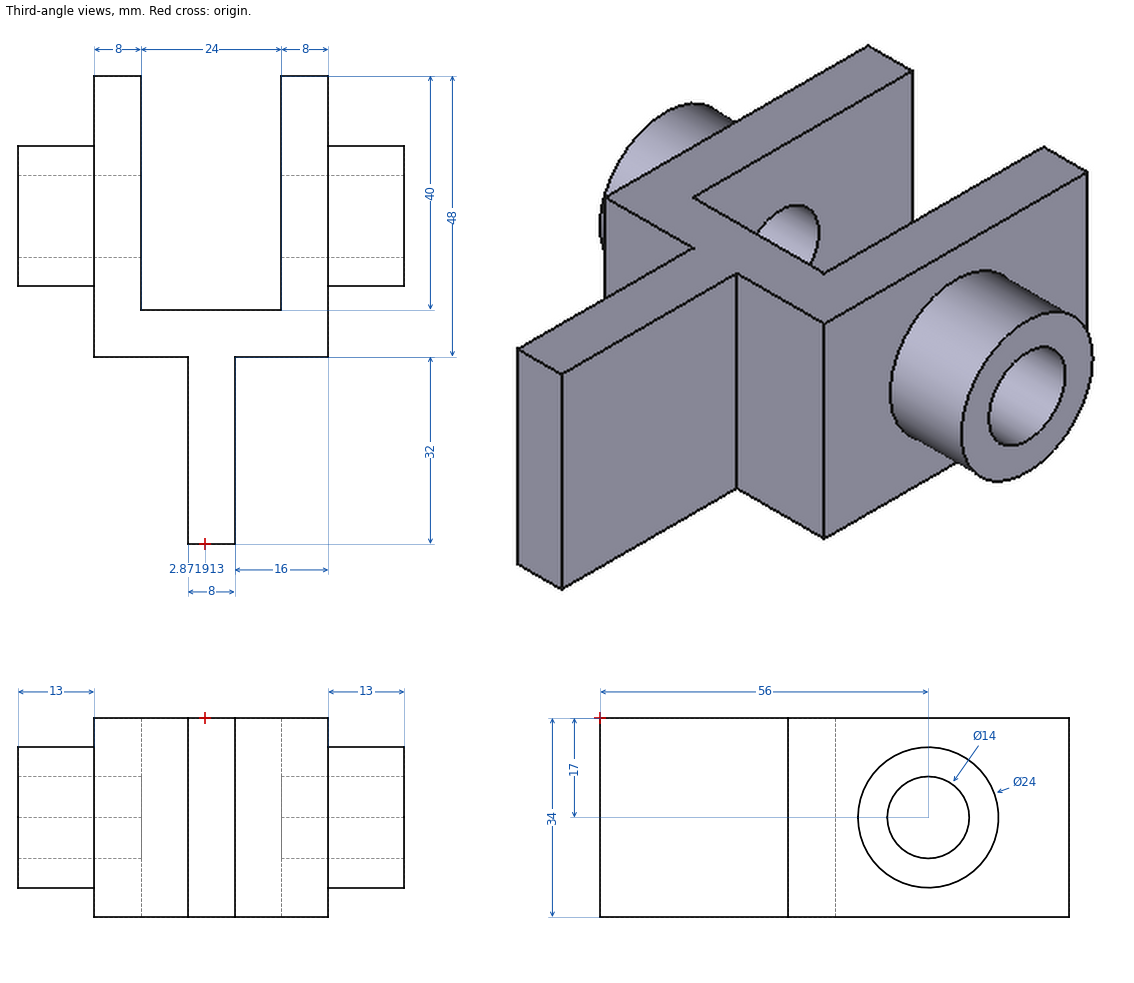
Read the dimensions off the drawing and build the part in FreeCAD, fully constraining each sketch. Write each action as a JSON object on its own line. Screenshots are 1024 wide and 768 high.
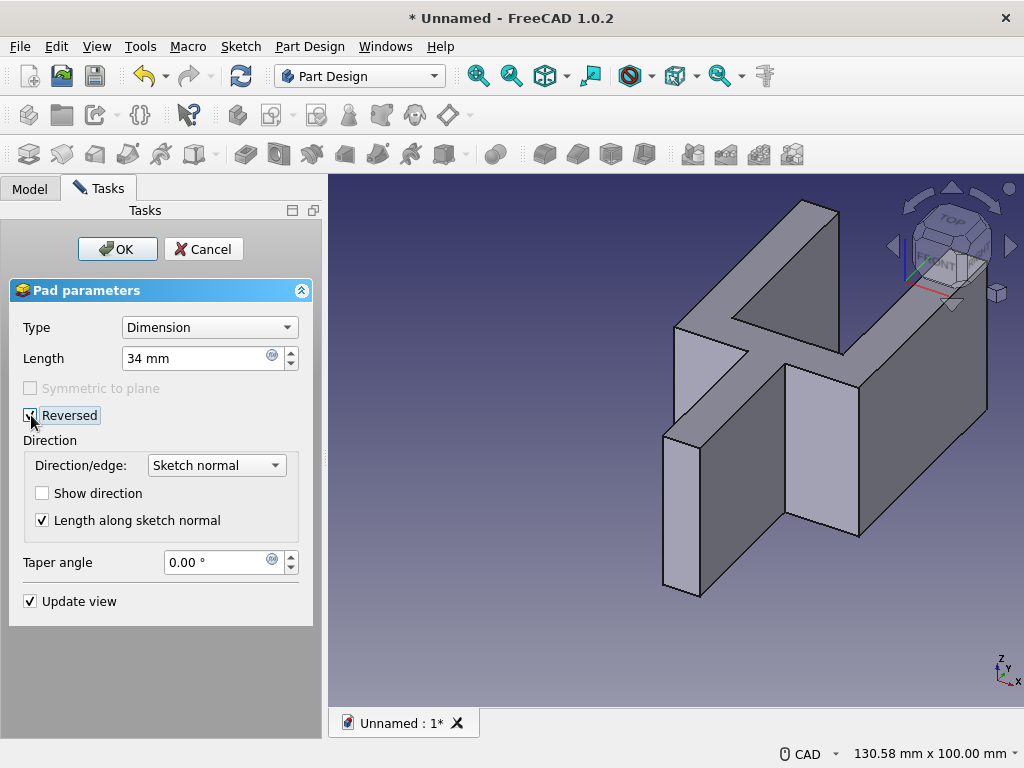
{"action": "left_click", "coordinate": [118, 249]}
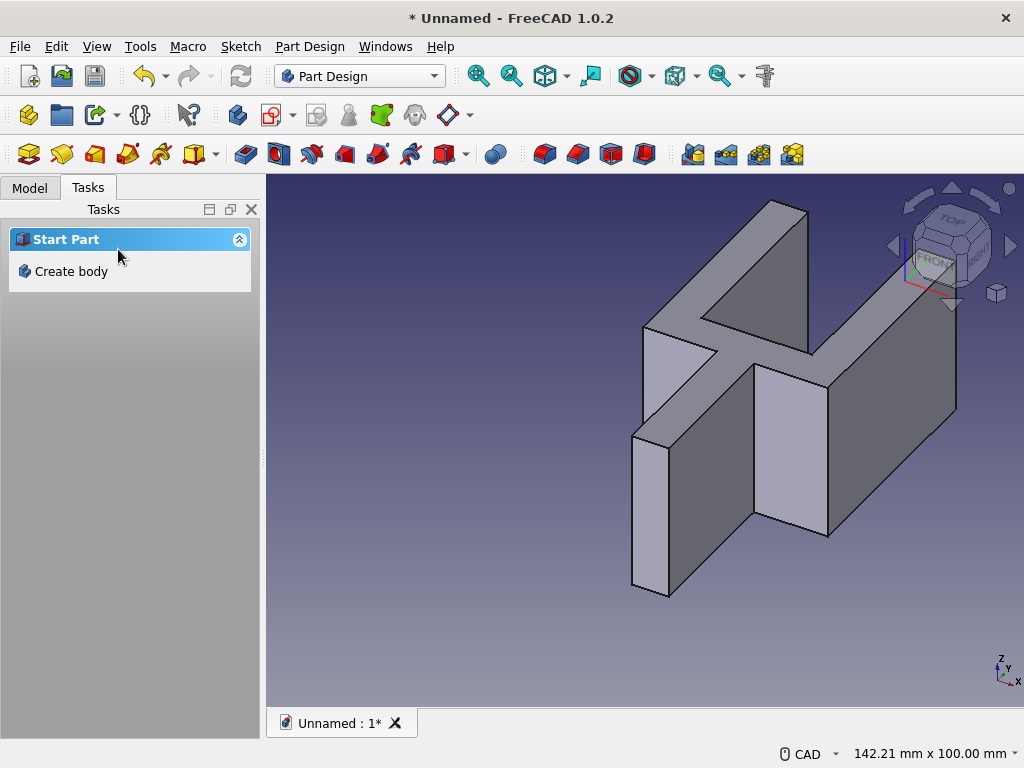
{"action": "left_click", "coordinate": [910, 380]}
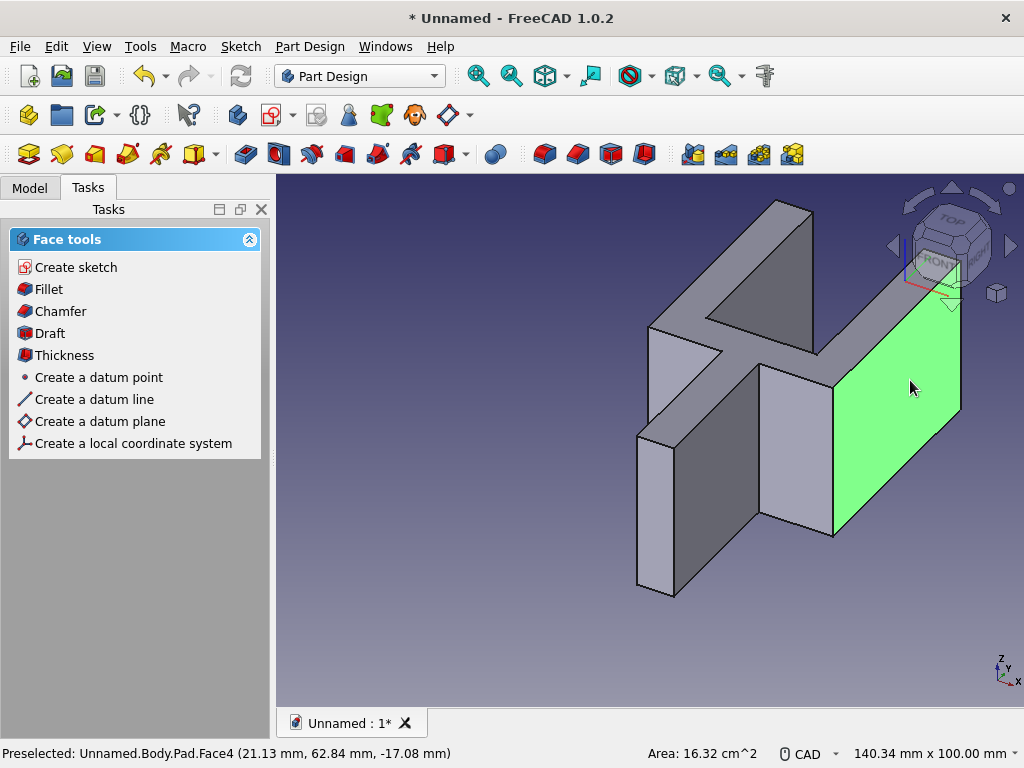
{"action": "left_click", "coordinate": [270, 116]}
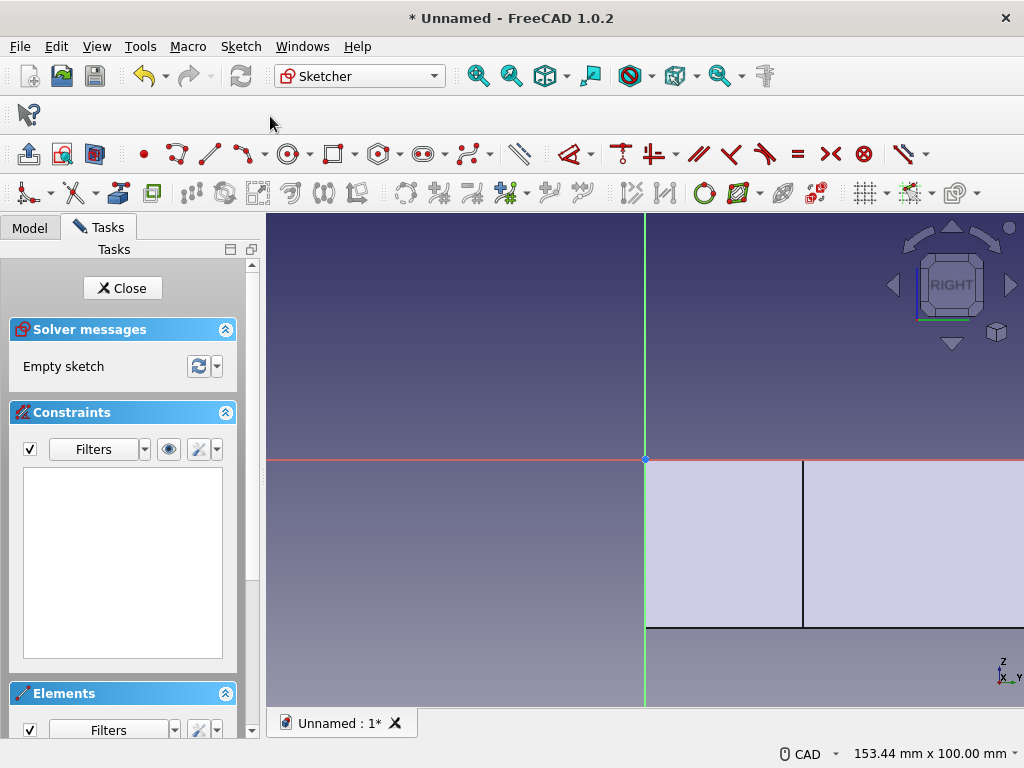
{"action": "scroll", "coordinate": [576, 460], "scroll_direction": "down", "scroll_amount": 5}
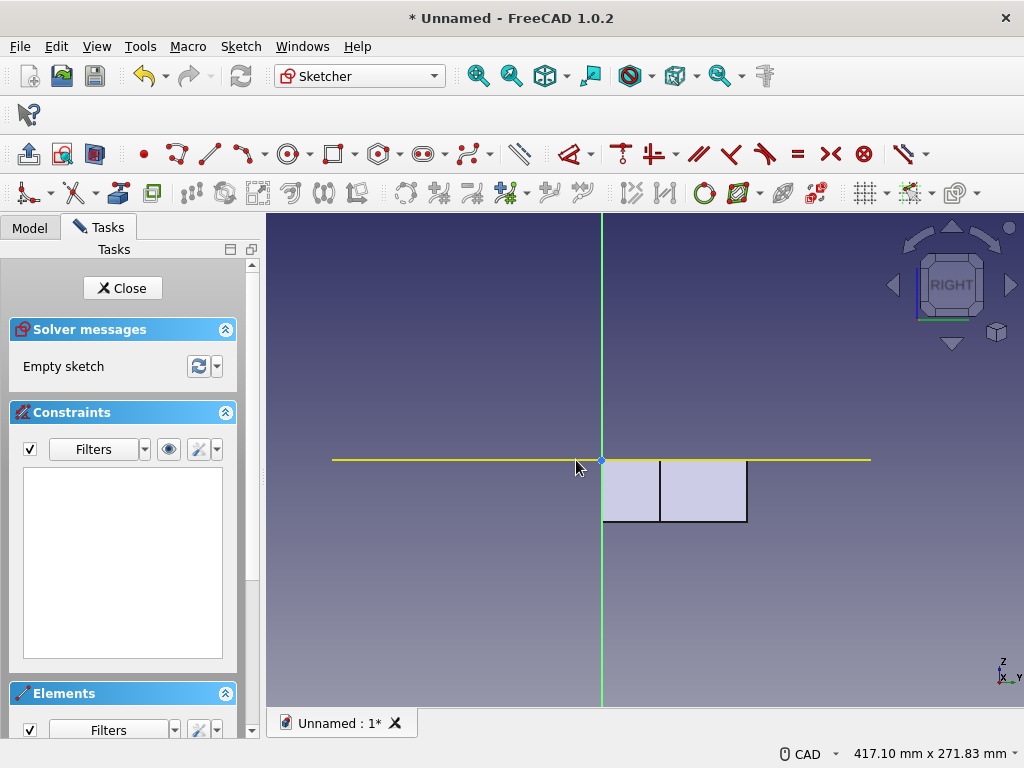
{"action": "scroll", "coordinate": [723, 496], "scroll_direction": "up", "scroll_amount": 10}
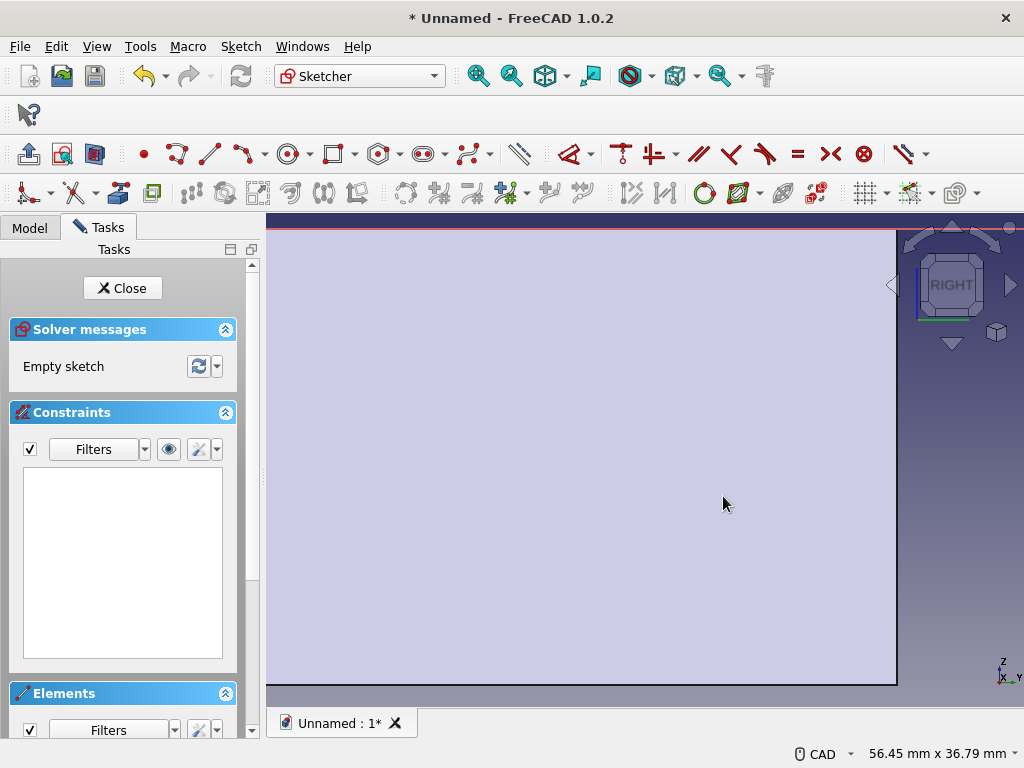
{"action": "left_click", "coordinate": [288, 154]}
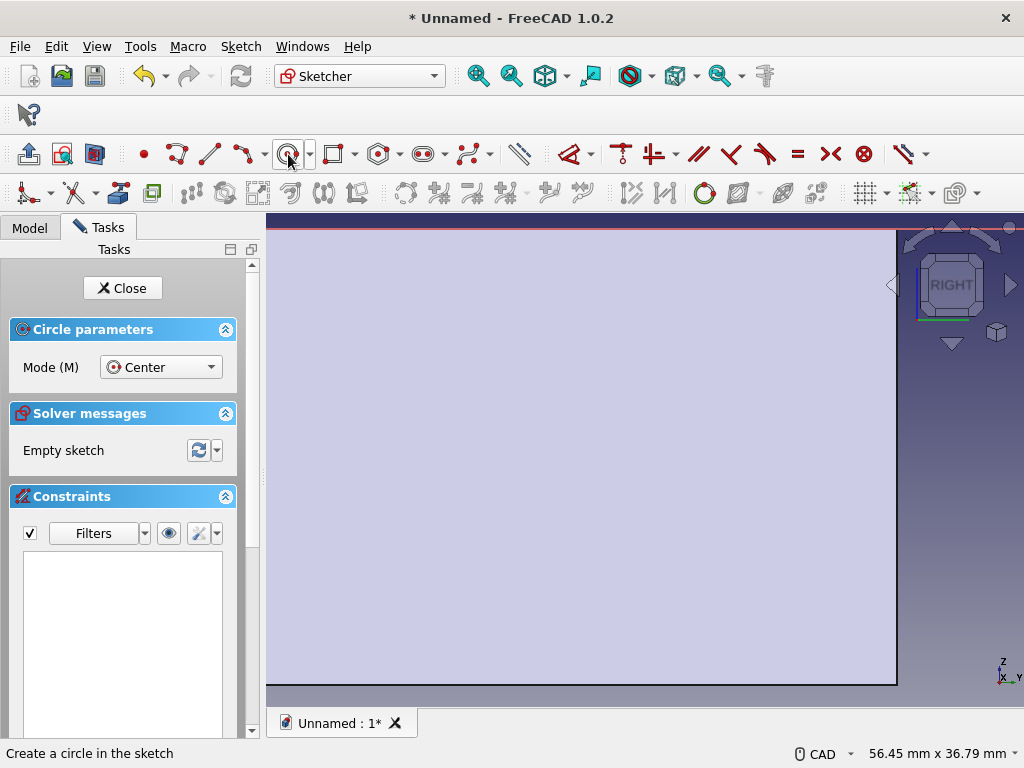
{"action": "left_click", "coordinate": [574, 457]}
{"action": "mouse_move", "coordinate": [688, 343]}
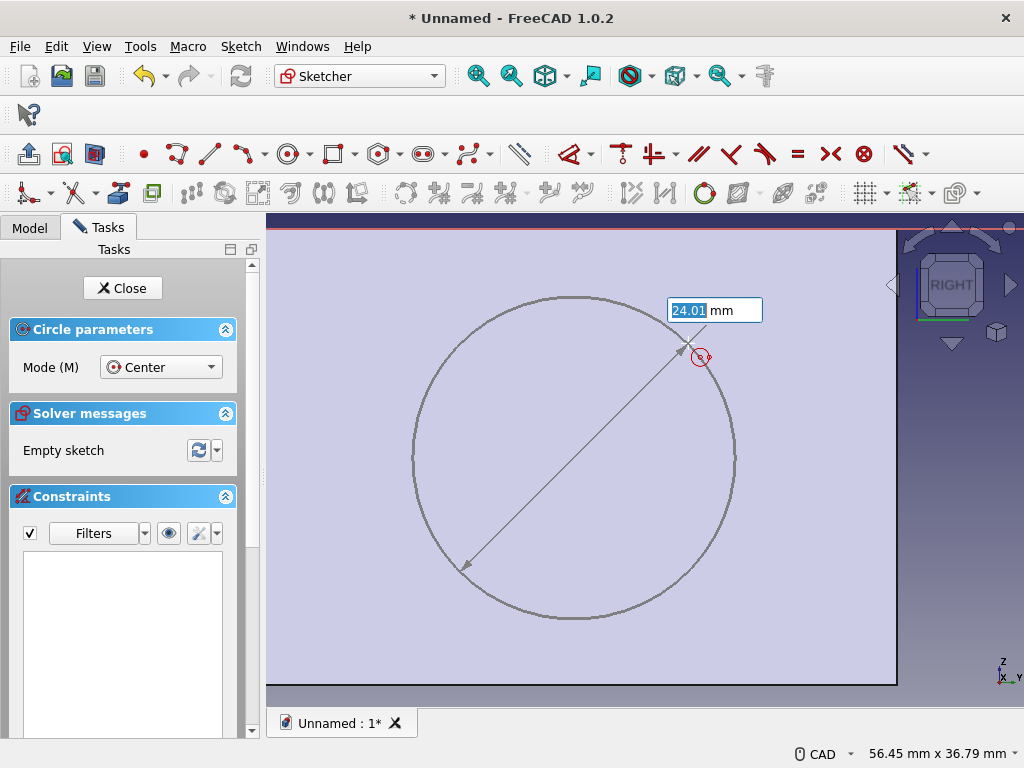
{"action": "type", "text": "24"}
{"action": "key", "text": "Return"}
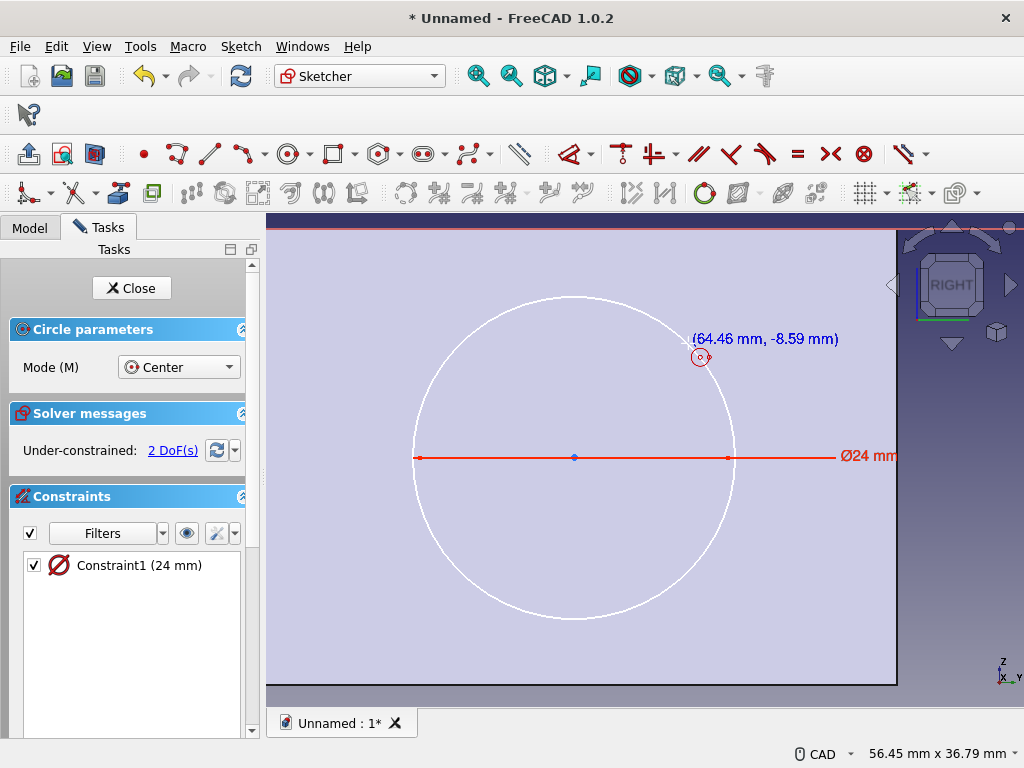
{"action": "left_click", "coordinate": [574, 458]}
{"action": "mouse_move", "coordinate": [641, 390]}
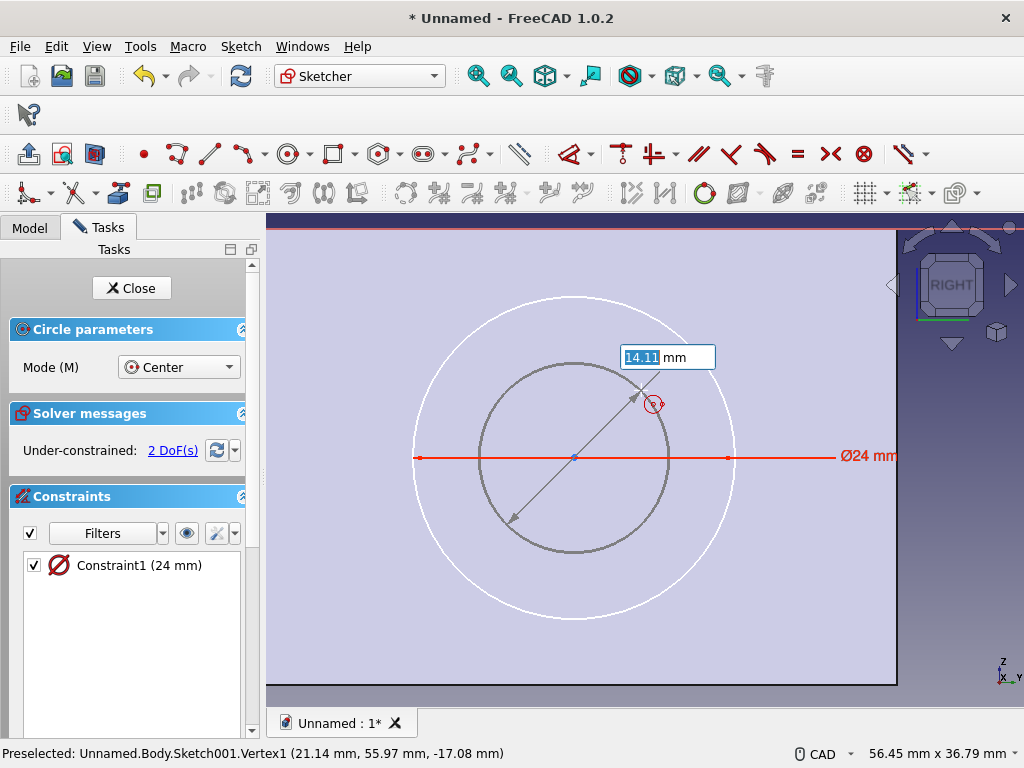
{"action": "type", "text": "14"}
{"action": "key", "text": "Return"}
{"action": "key", "text": "Escape"}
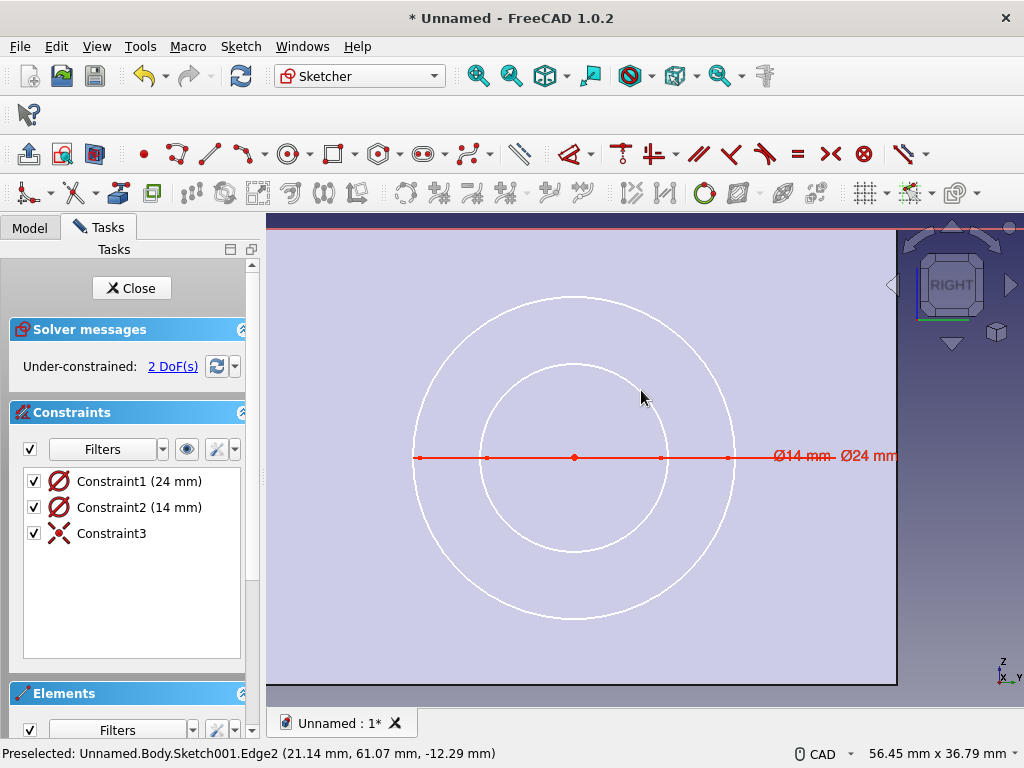
{"action": "key", "text": "d"}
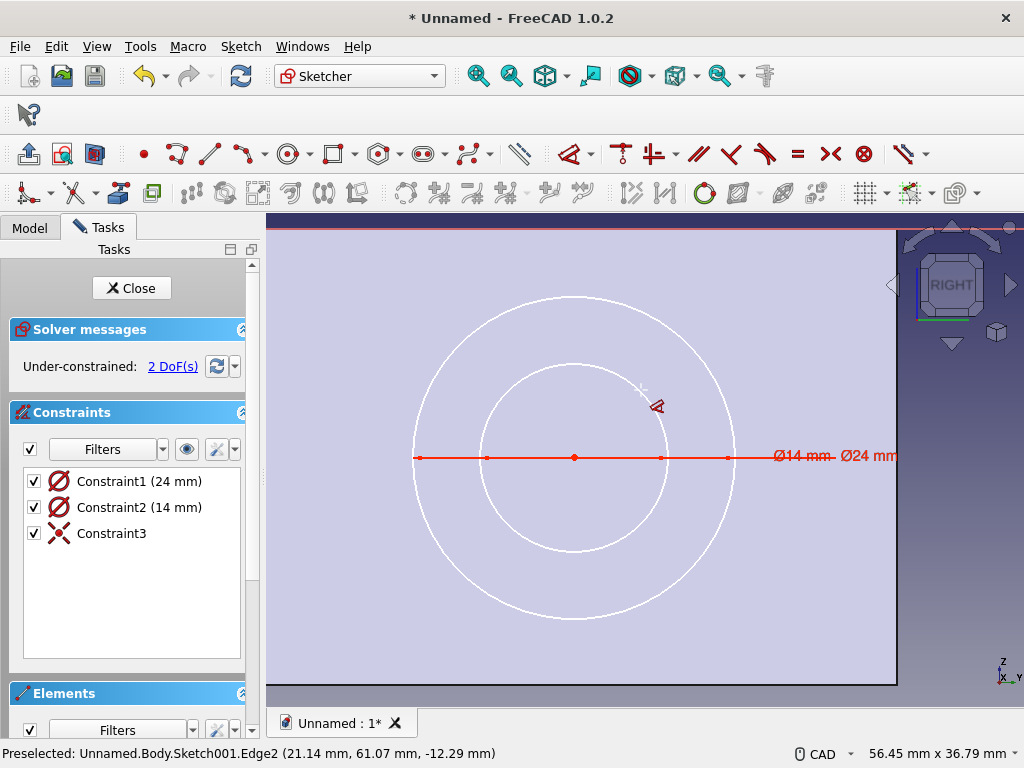
{"action": "left_click", "coordinate": [574, 458]}
{"action": "left_click", "coordinate": [434, 492]}